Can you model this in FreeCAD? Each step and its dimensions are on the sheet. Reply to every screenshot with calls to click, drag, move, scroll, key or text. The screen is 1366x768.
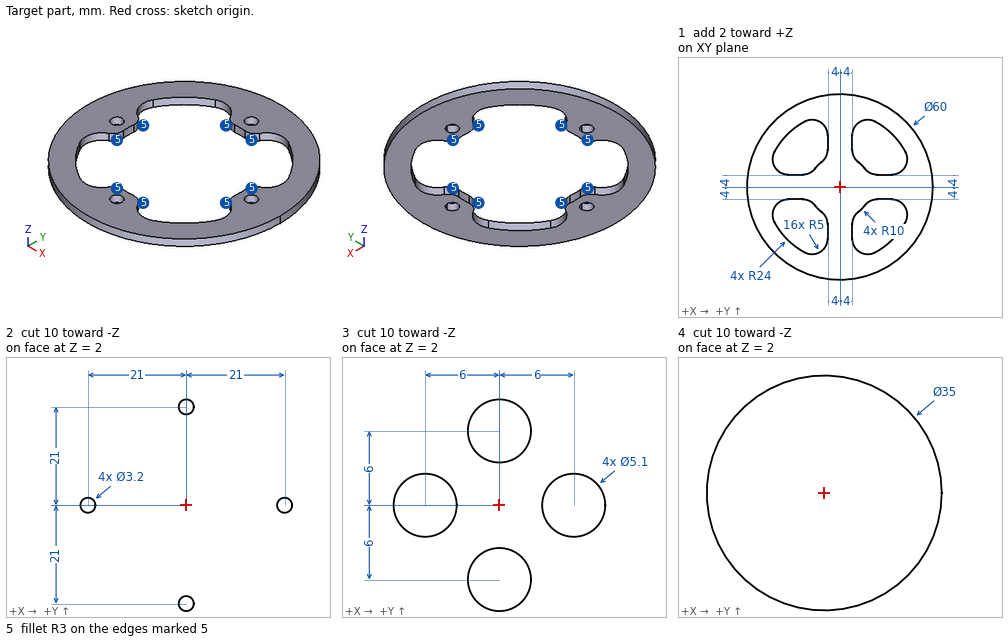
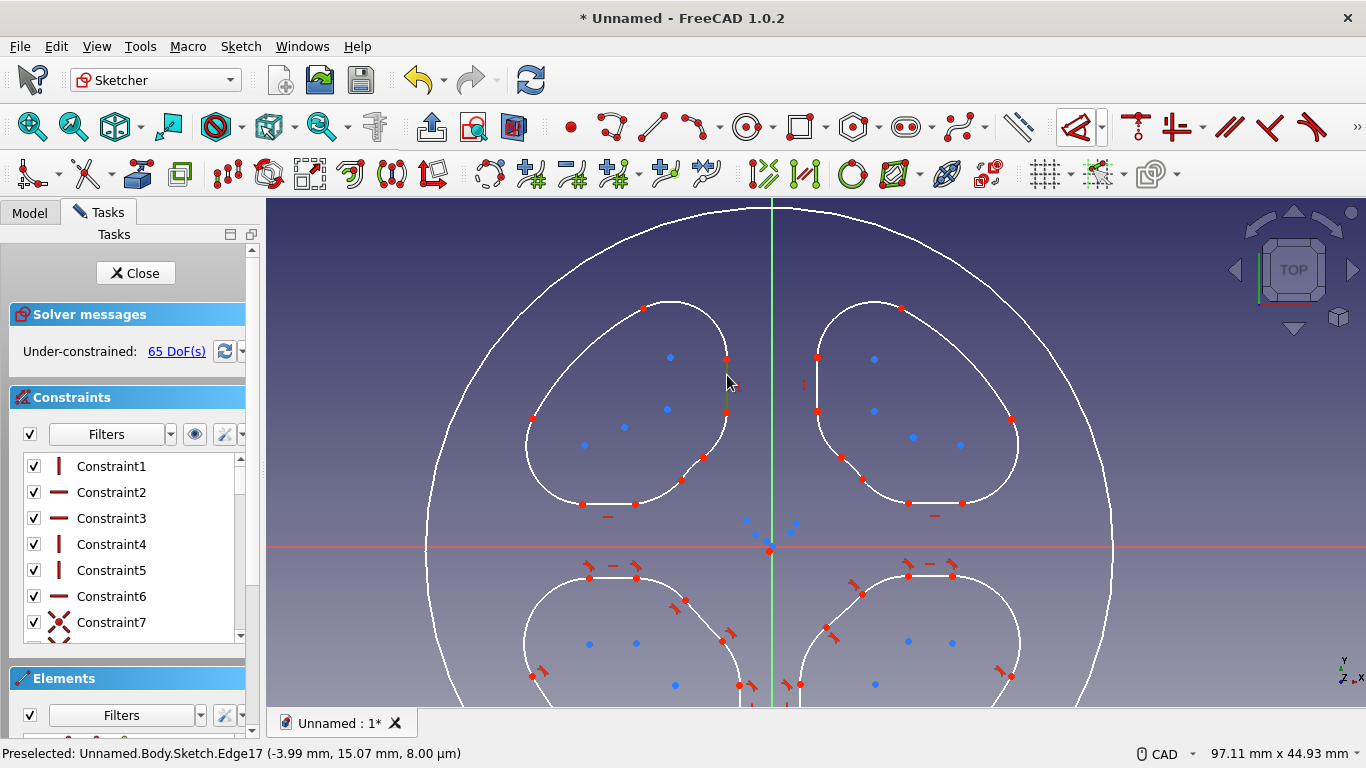
click(714, 446)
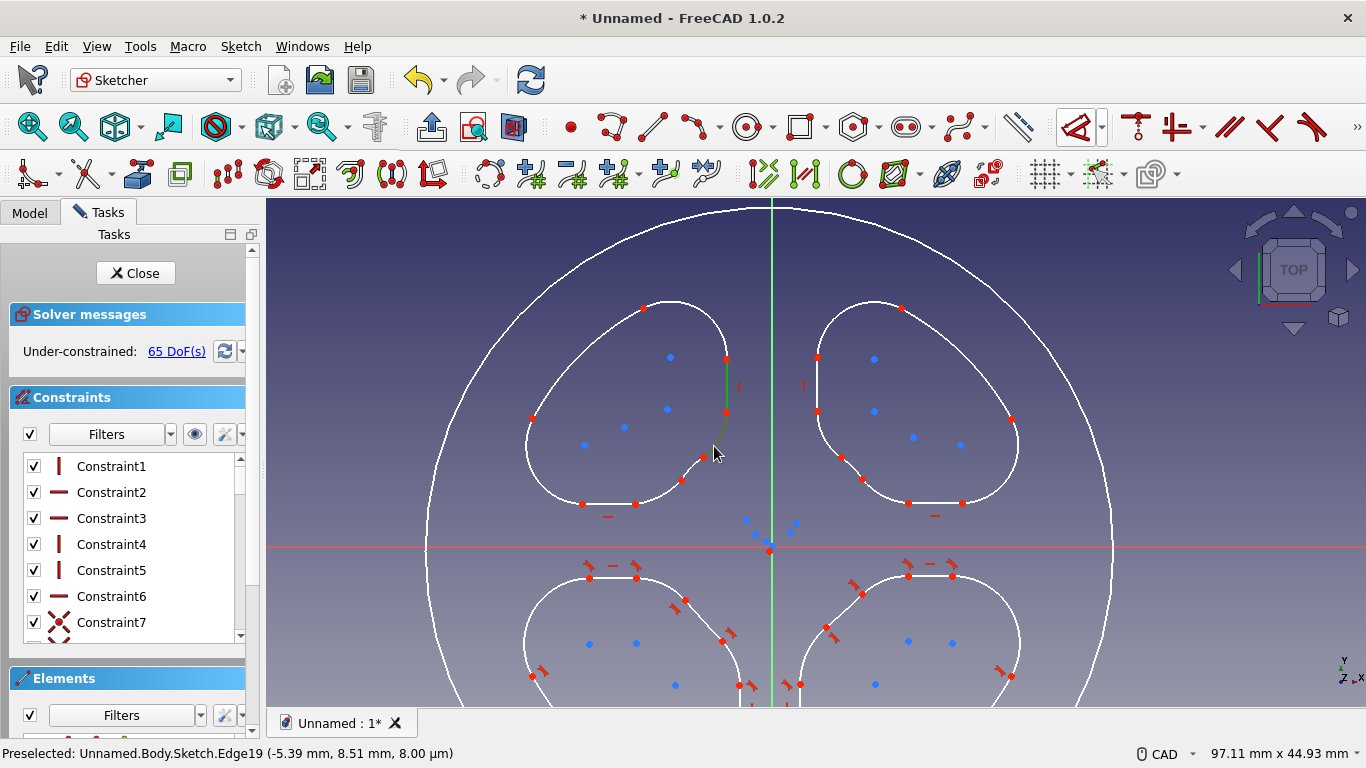
click(1312, 128)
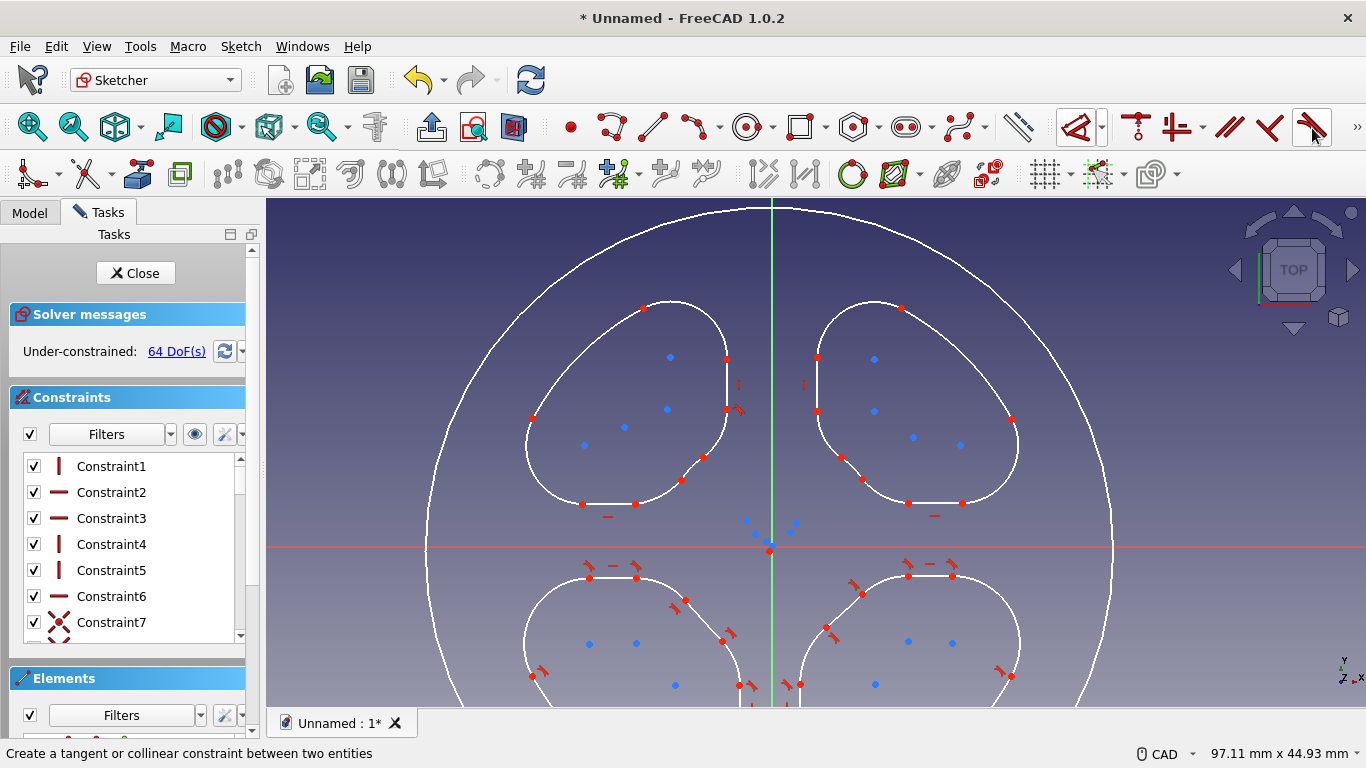
click(727, 374)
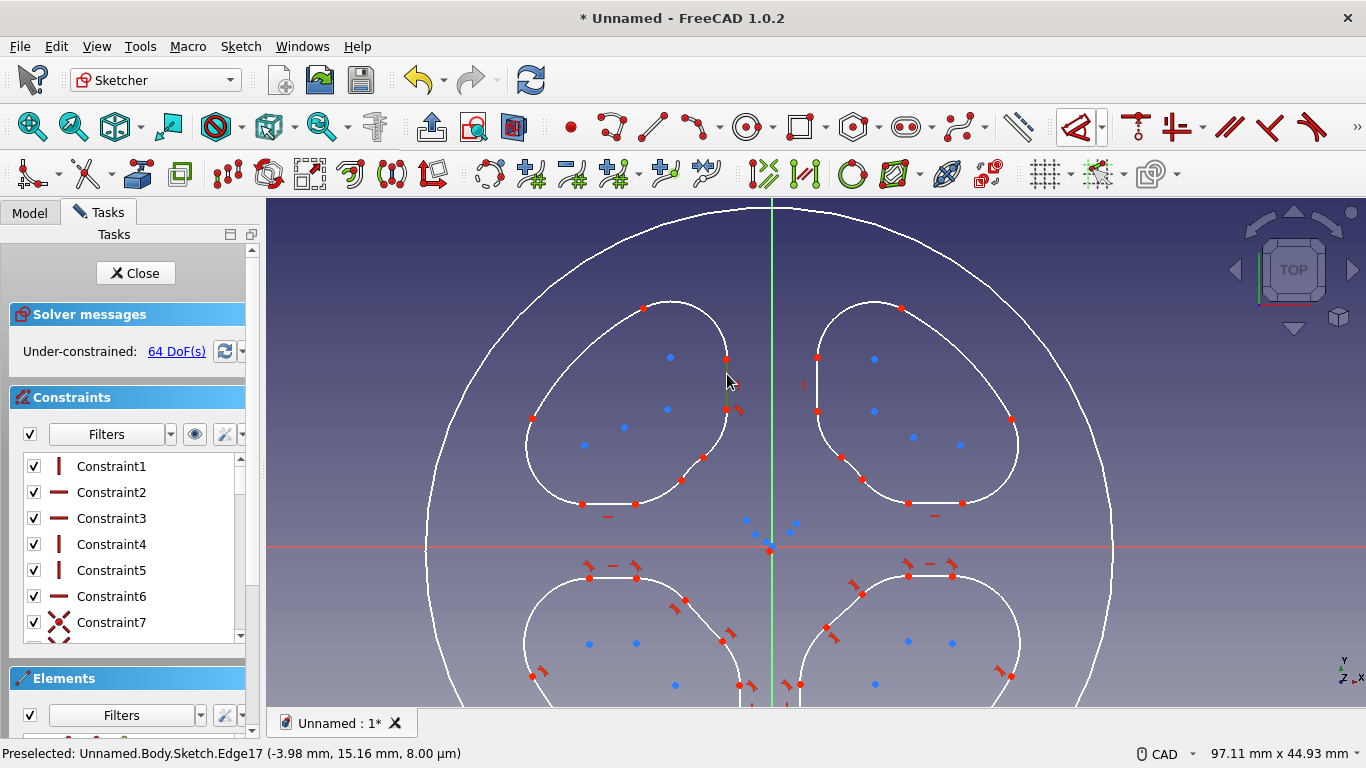
click(717, 326)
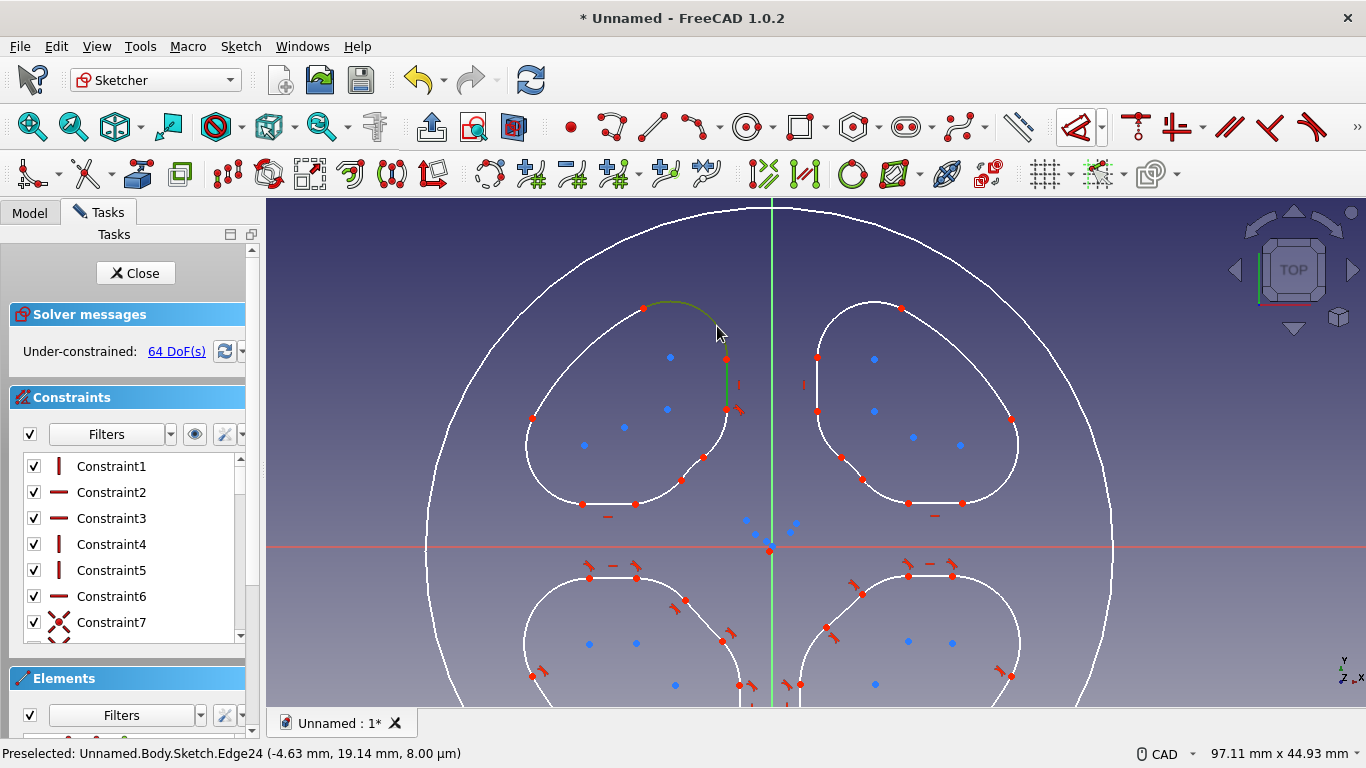
key(t)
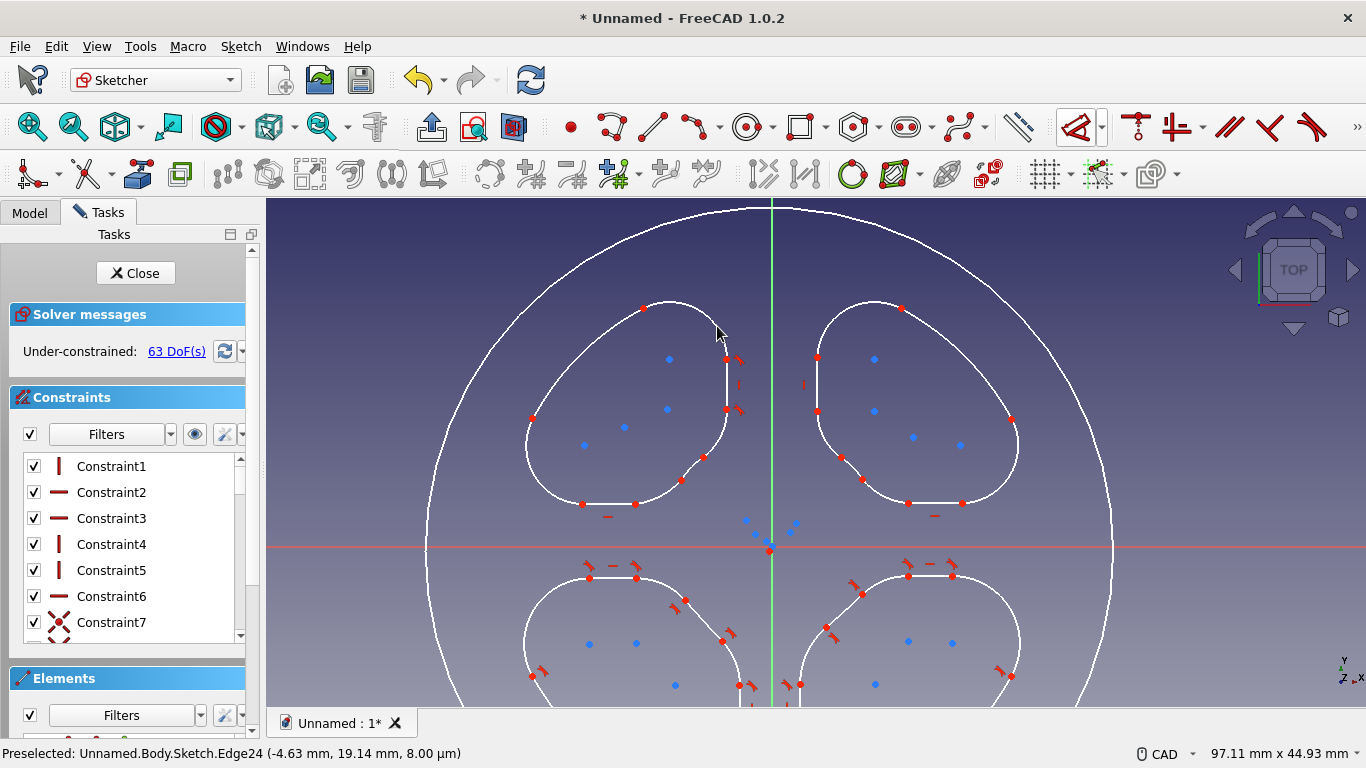
click(620, 504)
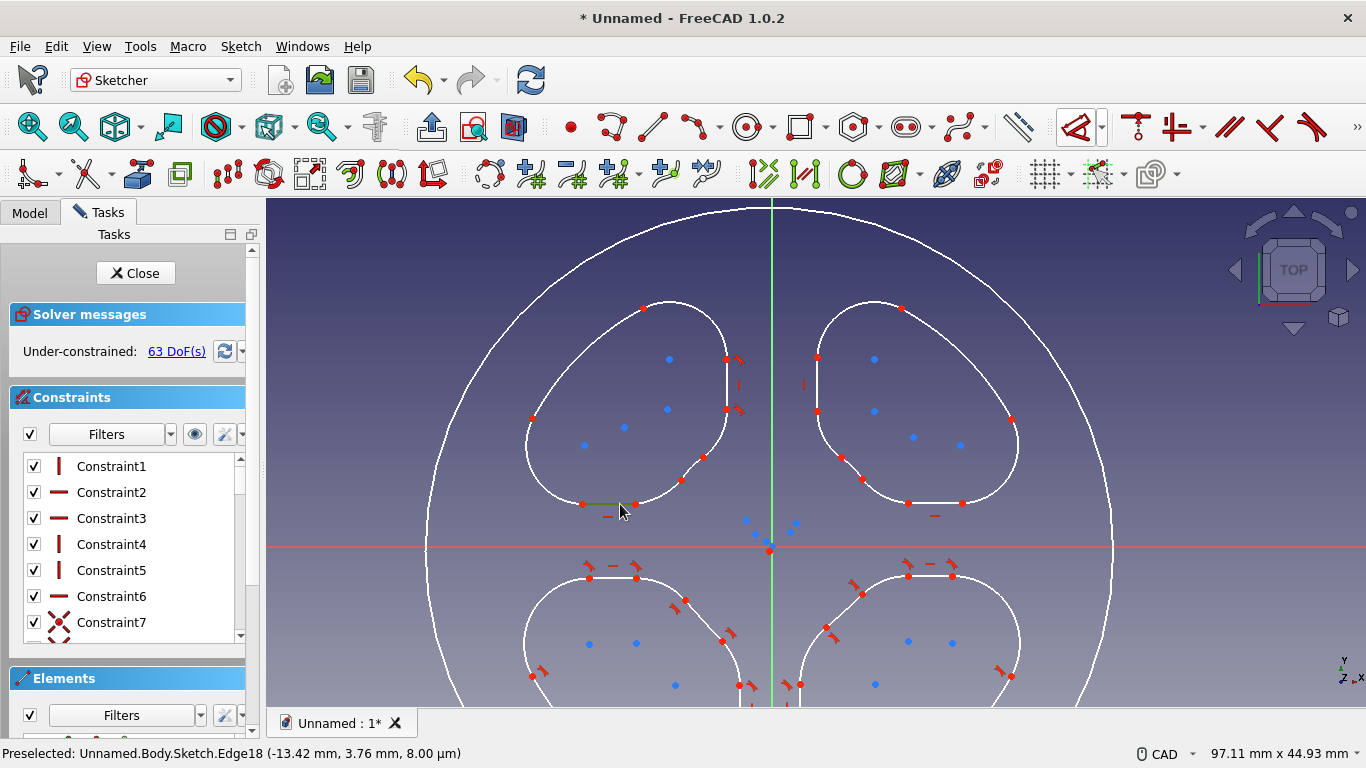
click(651, 500)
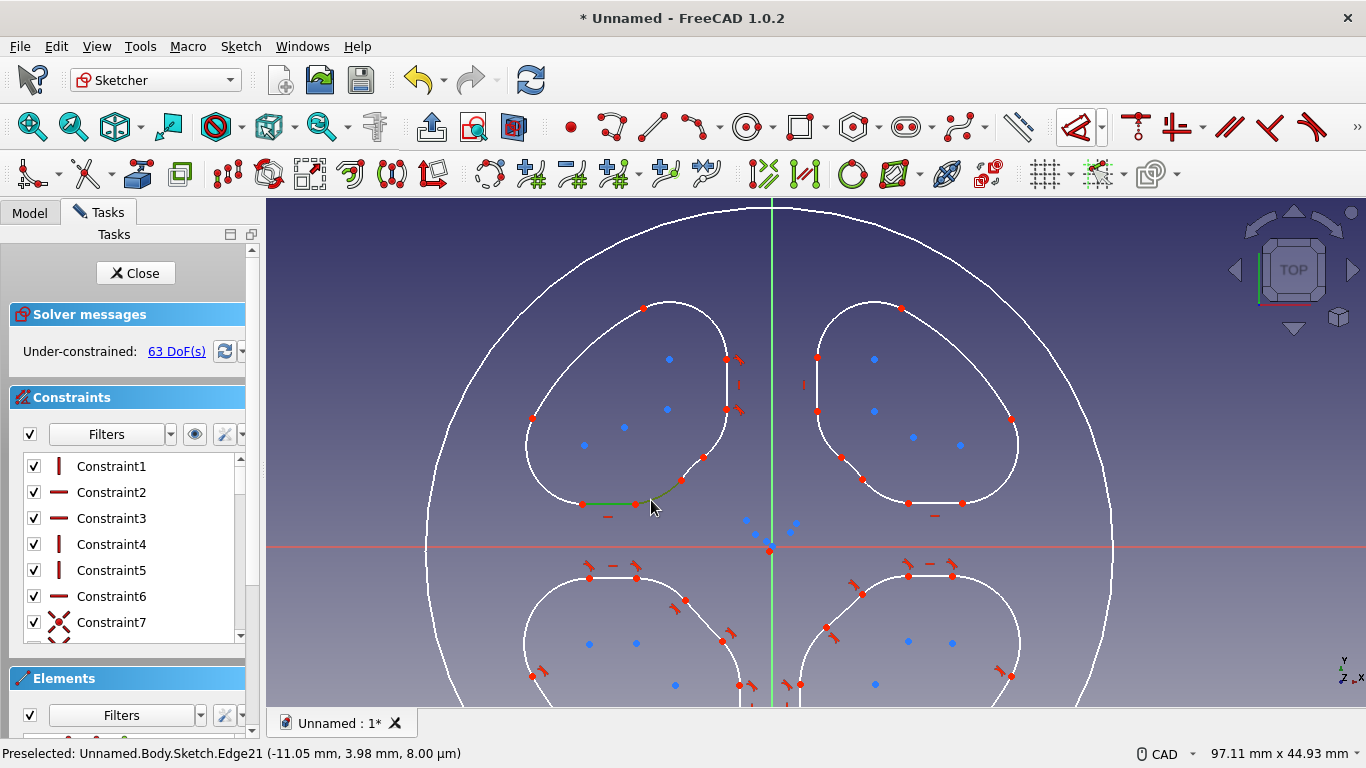
key(t)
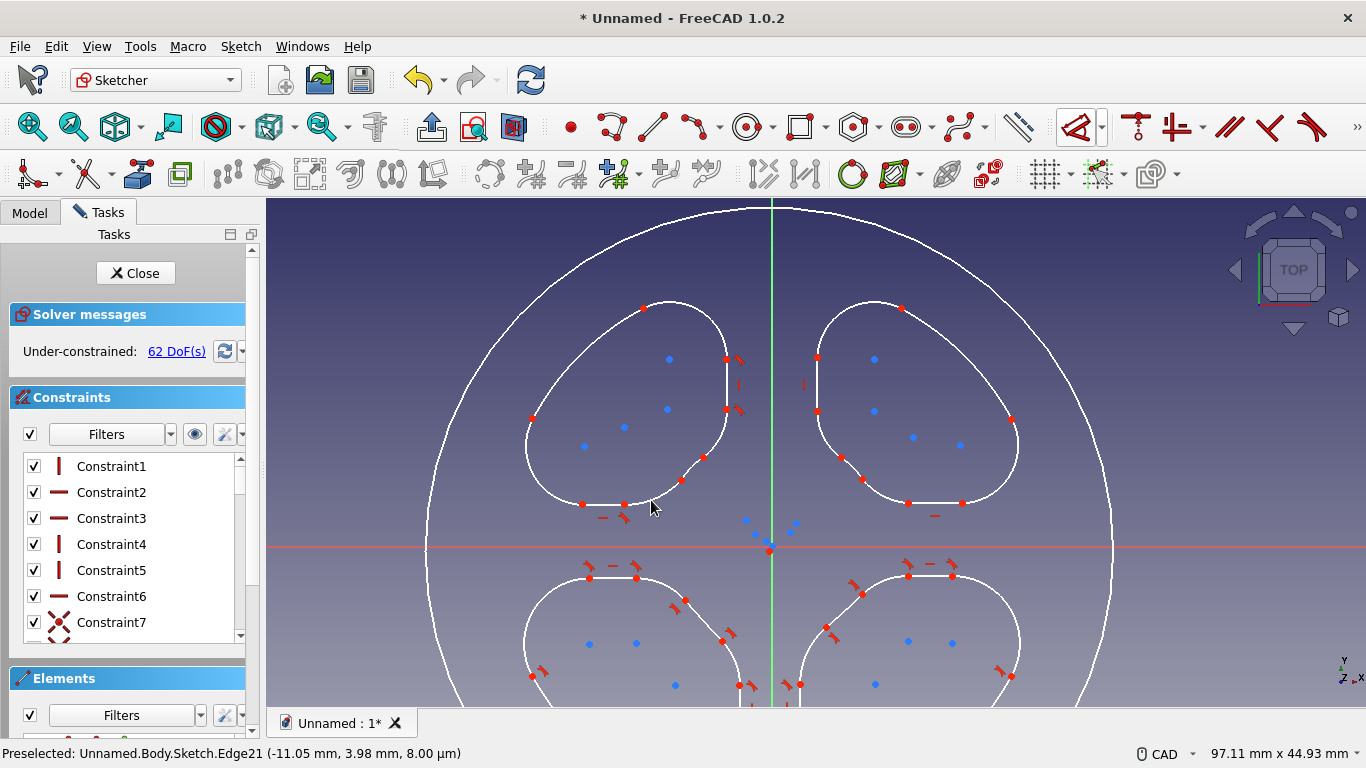
click(612, 505)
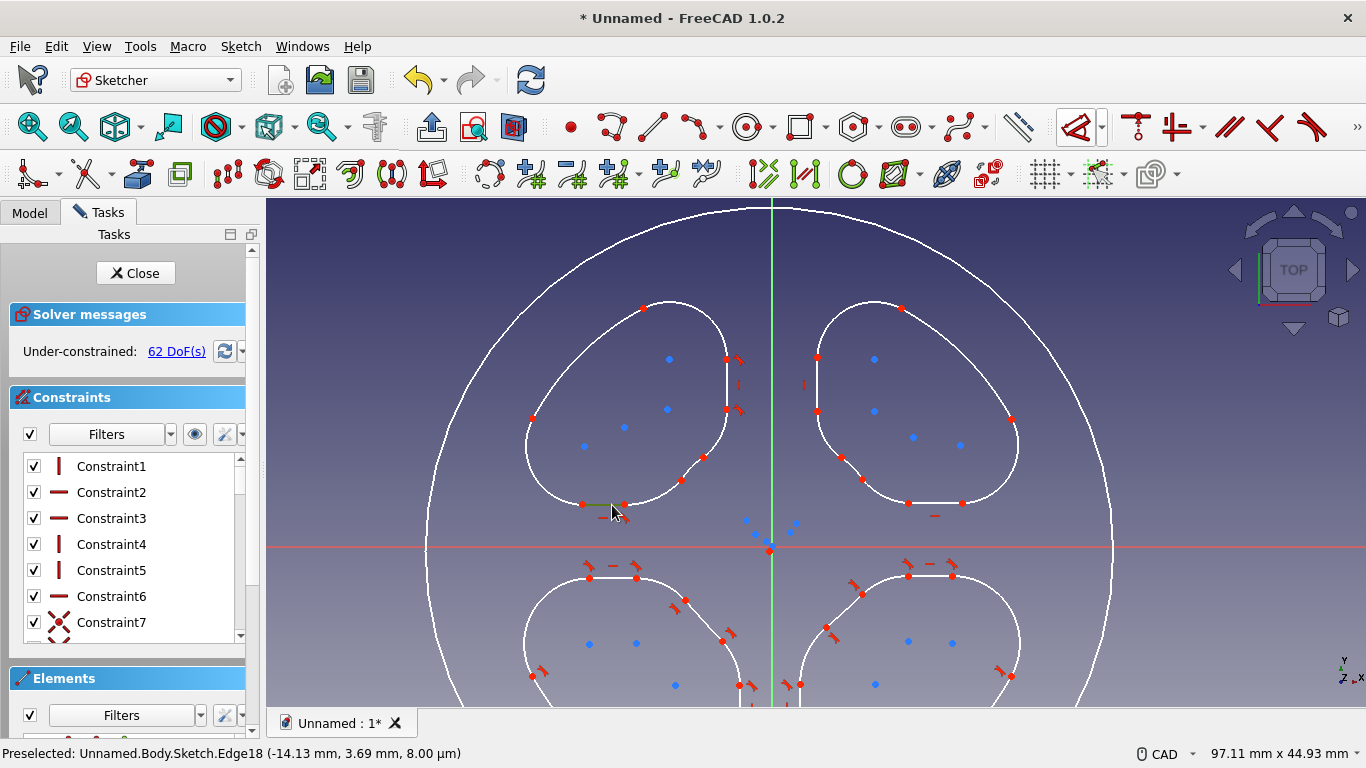
click(526, 453)